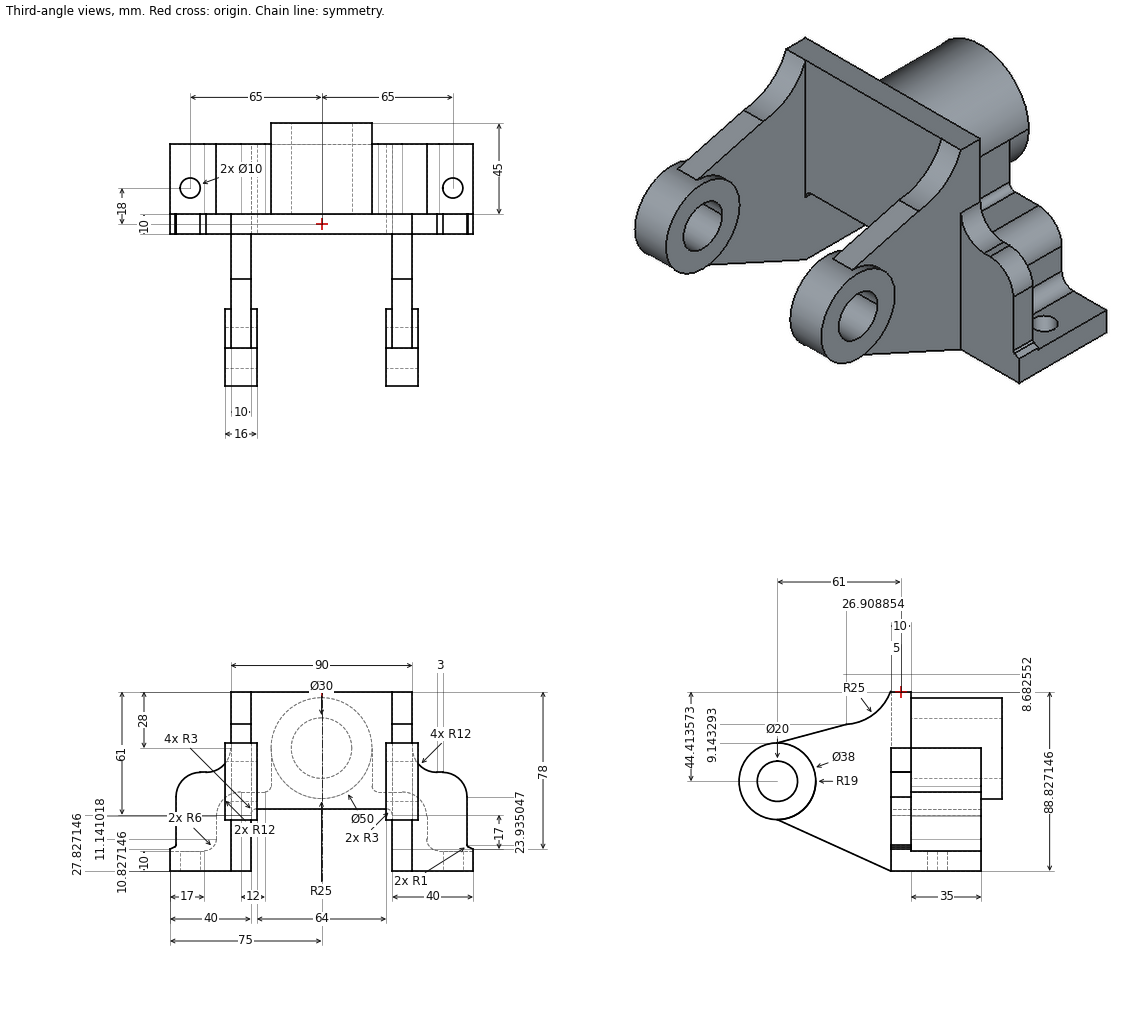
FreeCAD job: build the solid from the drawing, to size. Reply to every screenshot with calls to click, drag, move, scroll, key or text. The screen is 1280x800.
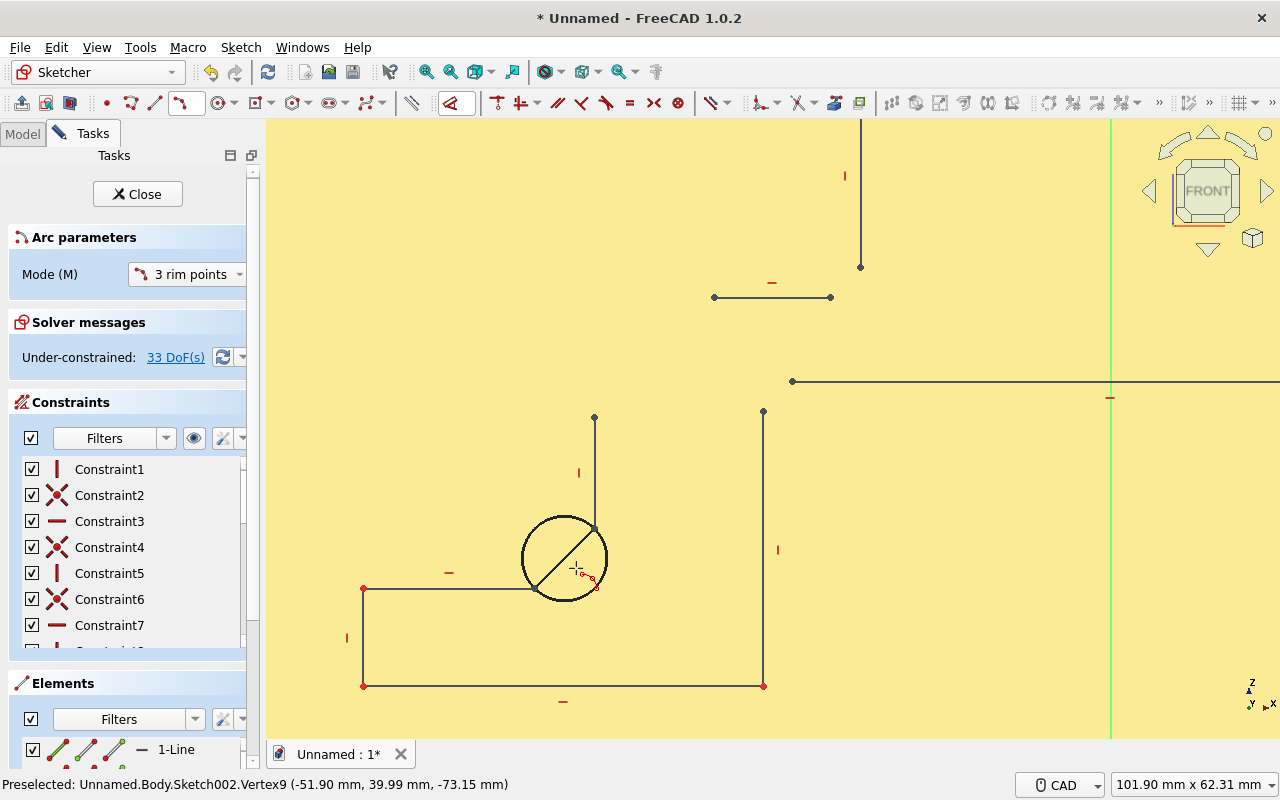
click(576, 568)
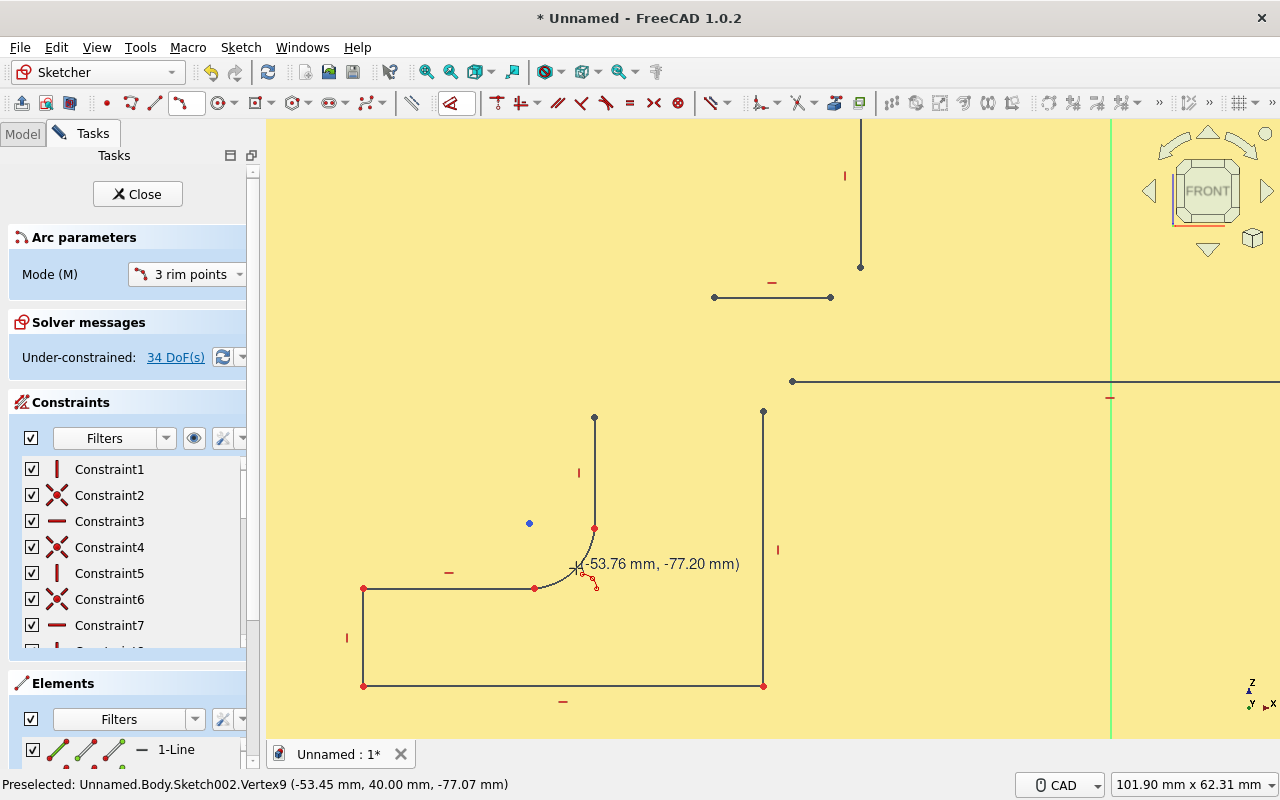
click(595, 417)
click(714, 298)
click(628, 330)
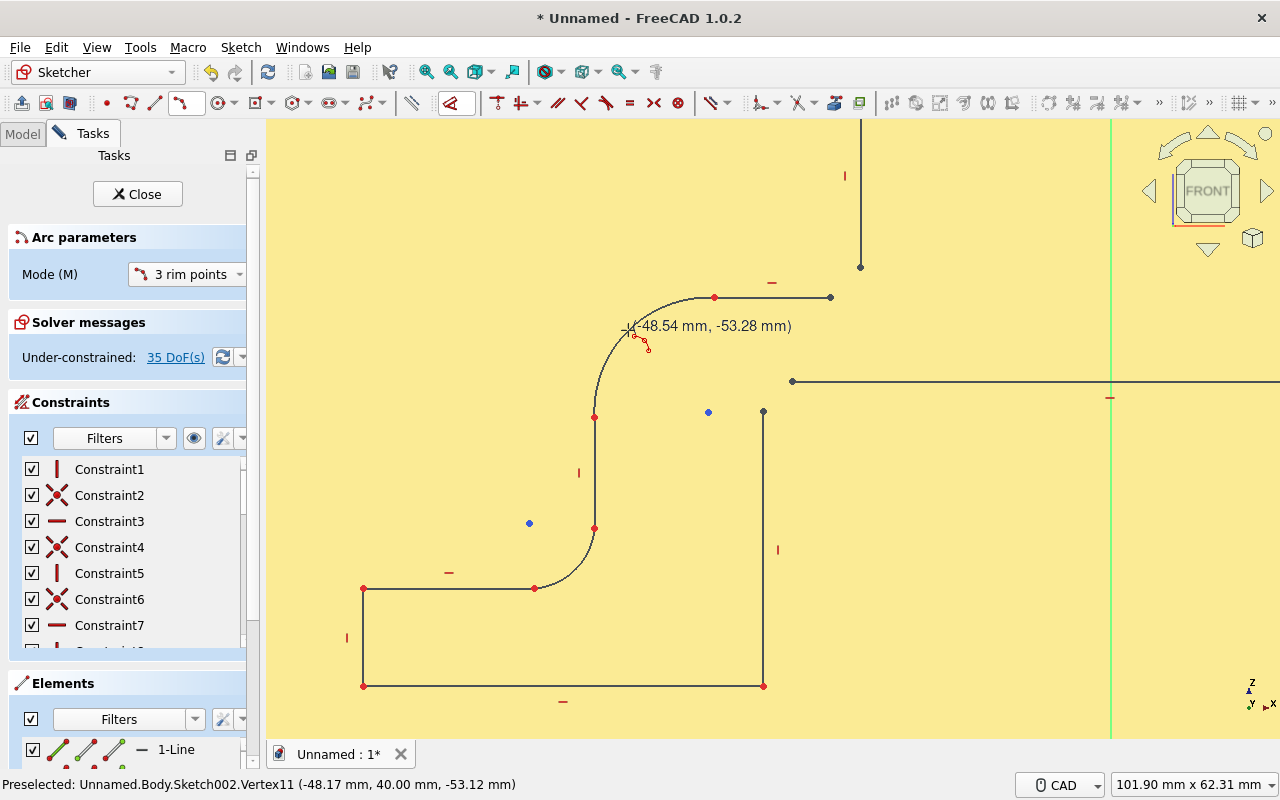
click(831, 298)
click(861, 268)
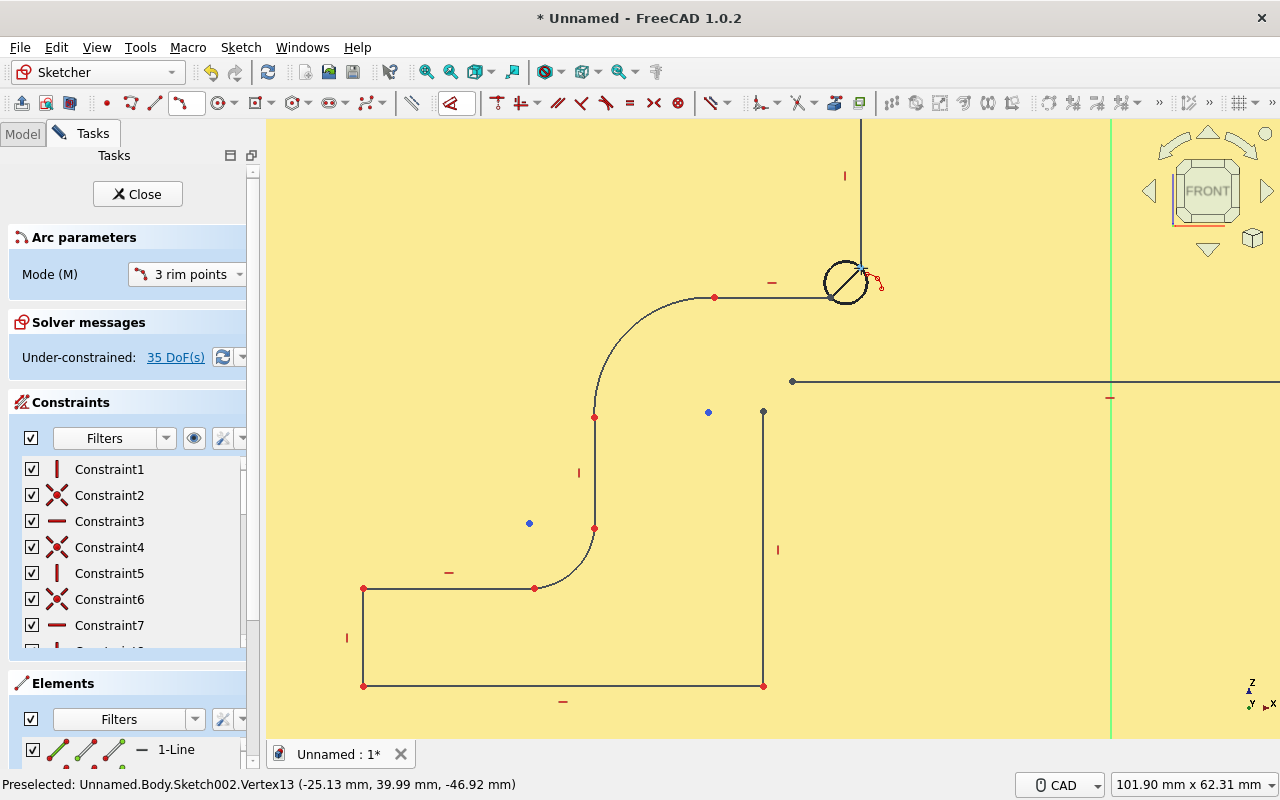
scroll(853, 287, up, 3)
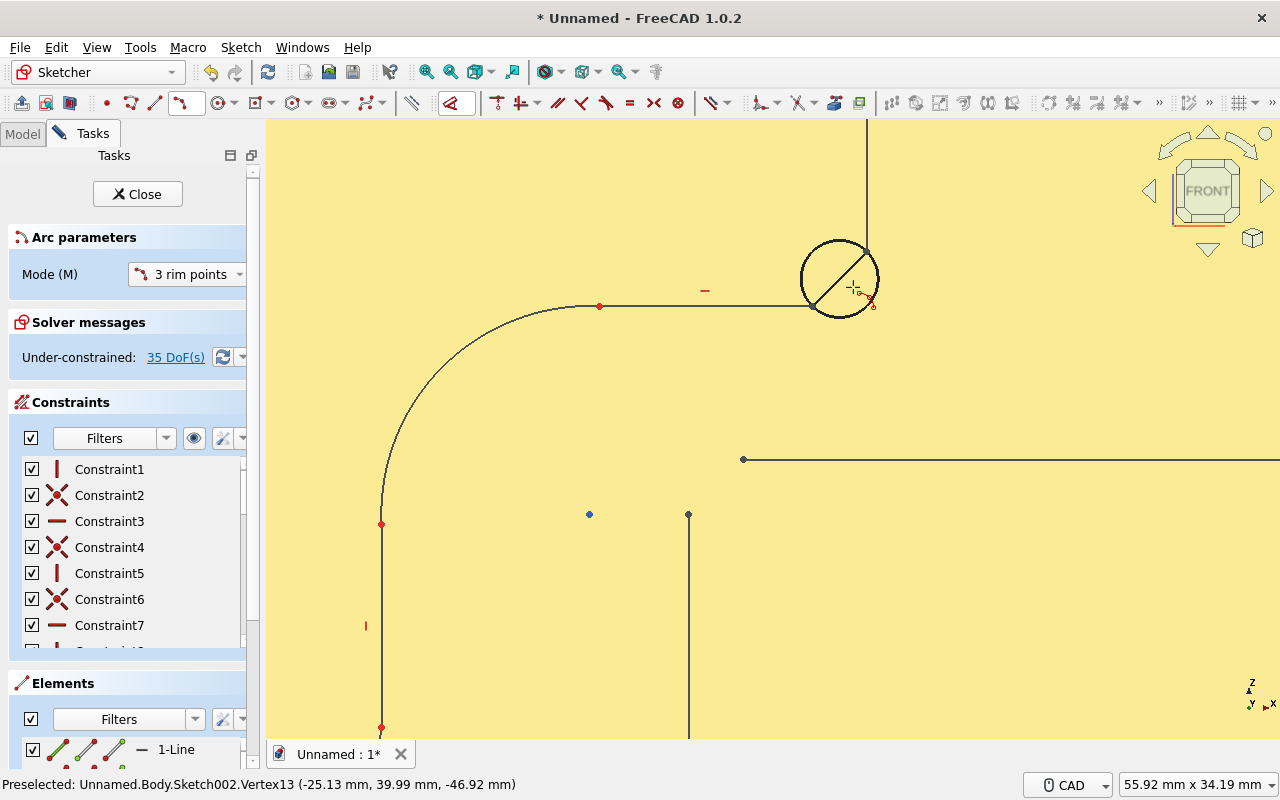
click(853, 286)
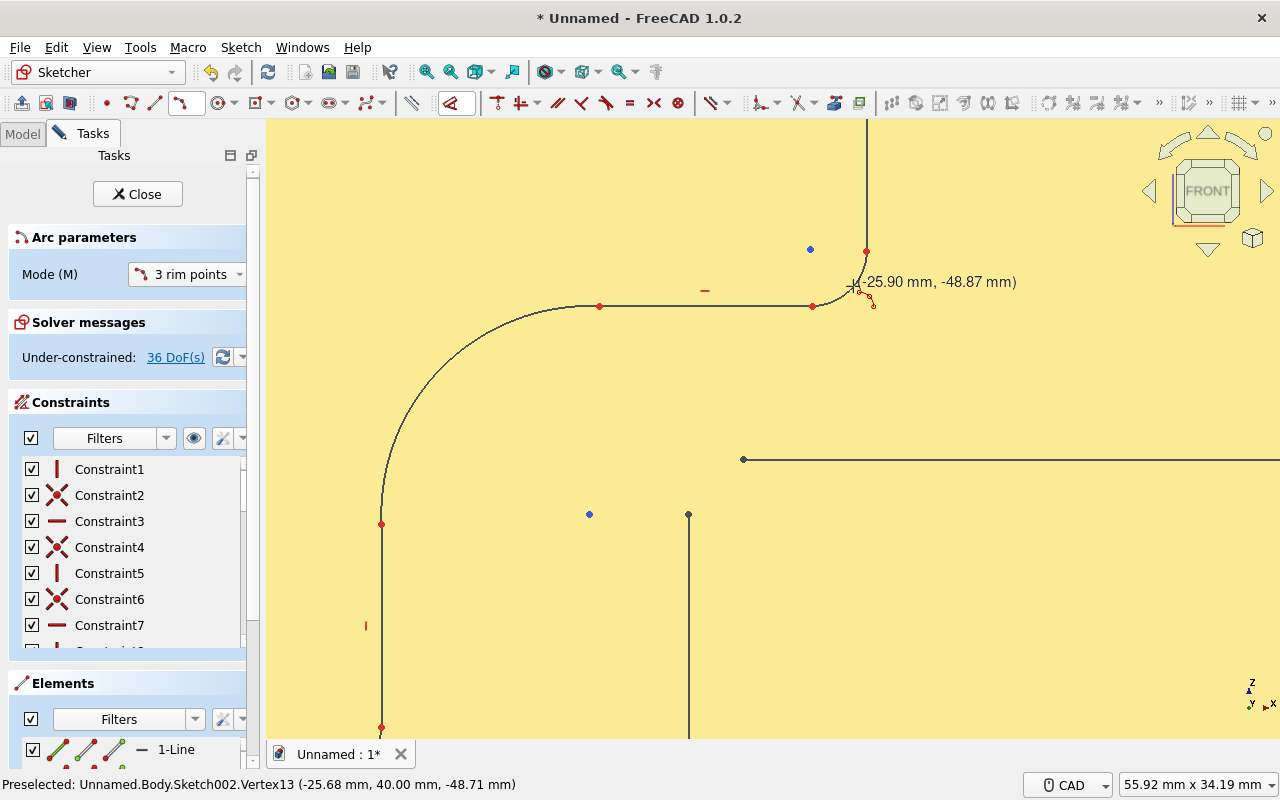
scroll(548, 485, down, 8)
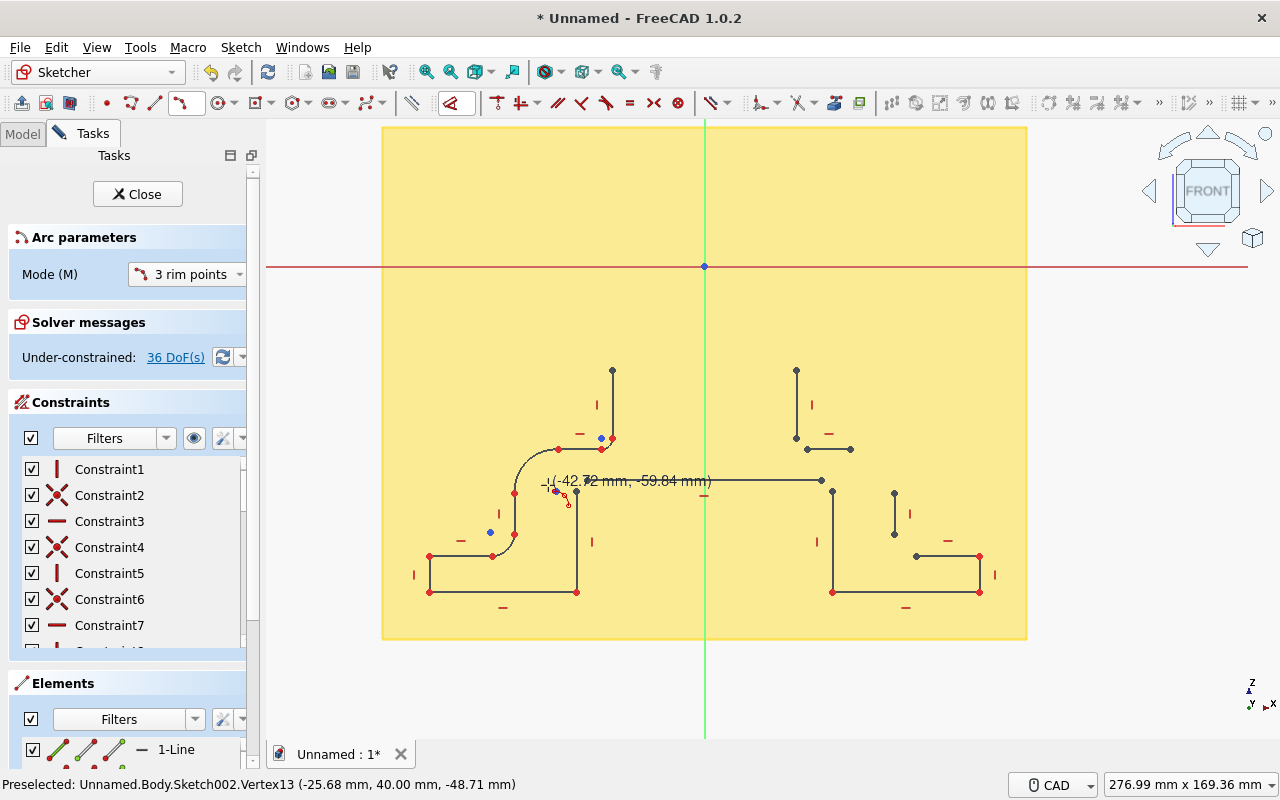
click(613, 370)
click(797, 370)
click(676, 456)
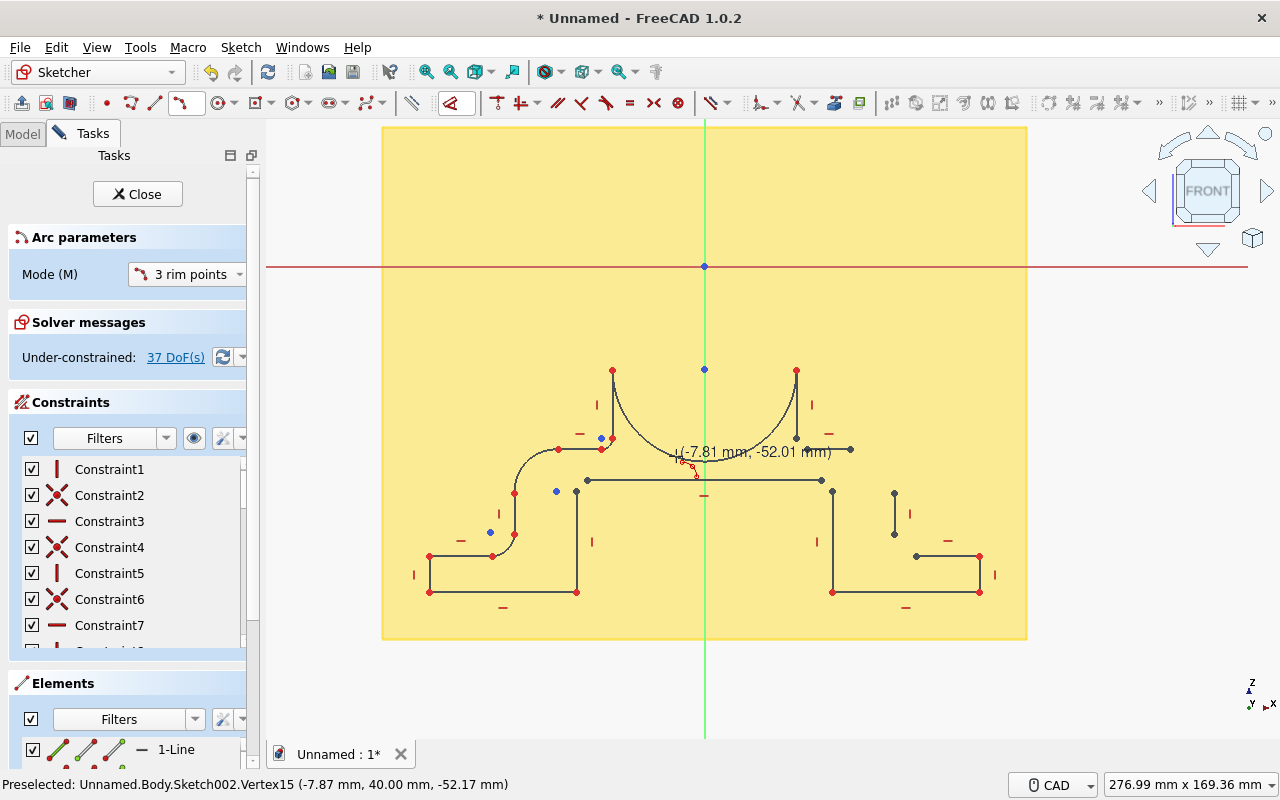
click(797, 438)
click(808, 449)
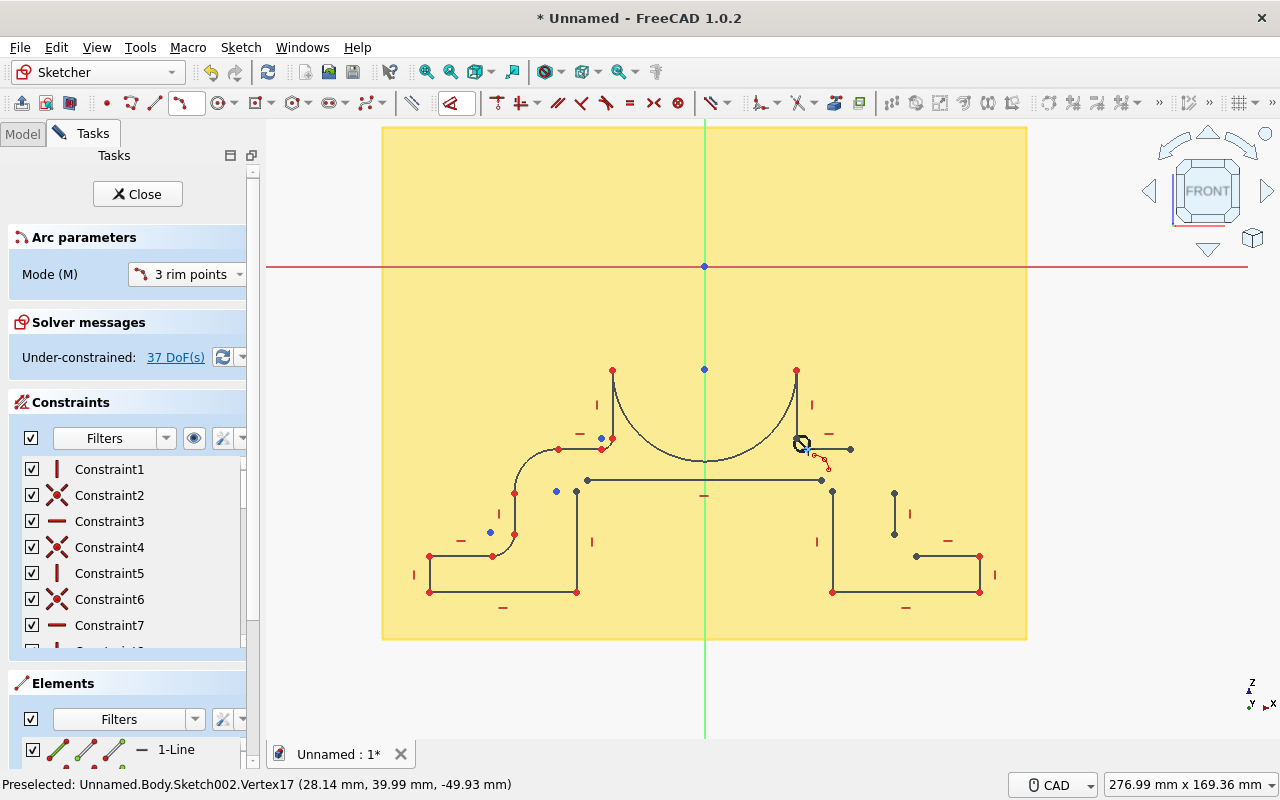
scroll(799, 445, up, 8)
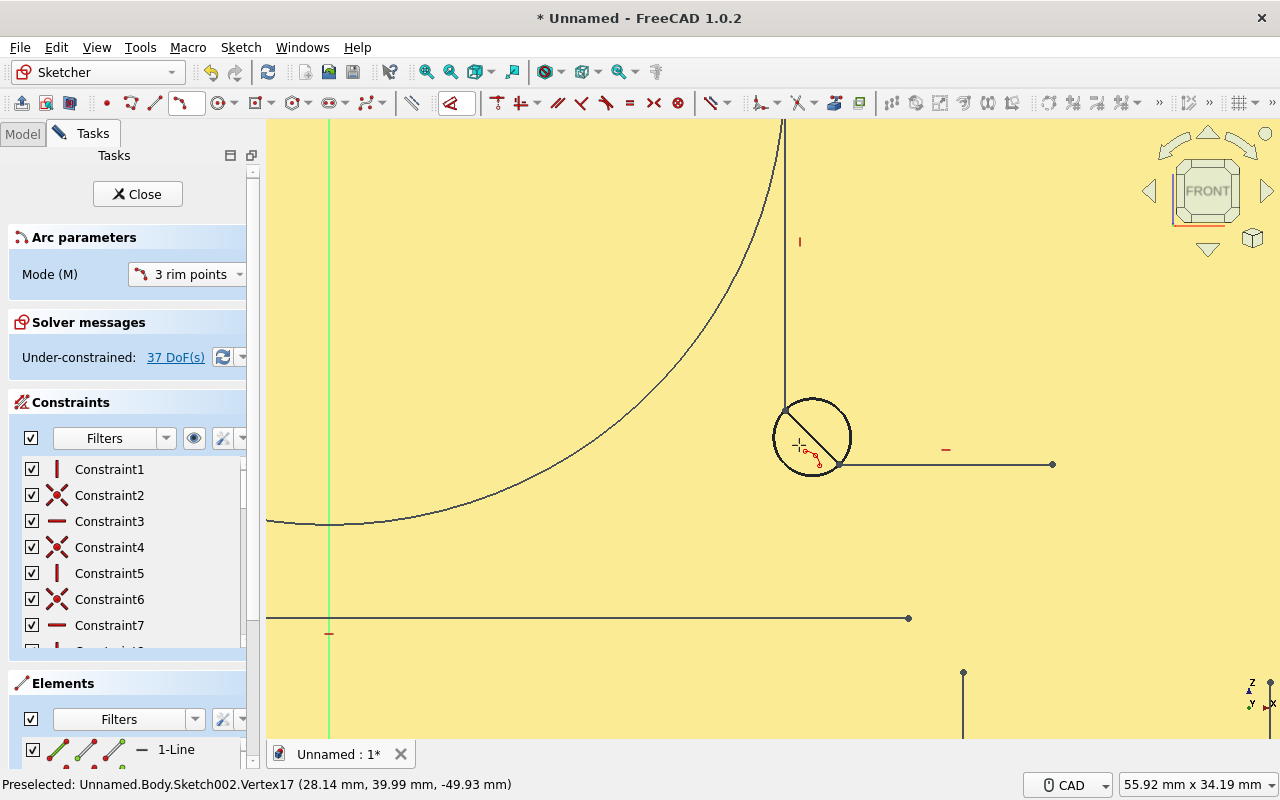
click(799, 444)